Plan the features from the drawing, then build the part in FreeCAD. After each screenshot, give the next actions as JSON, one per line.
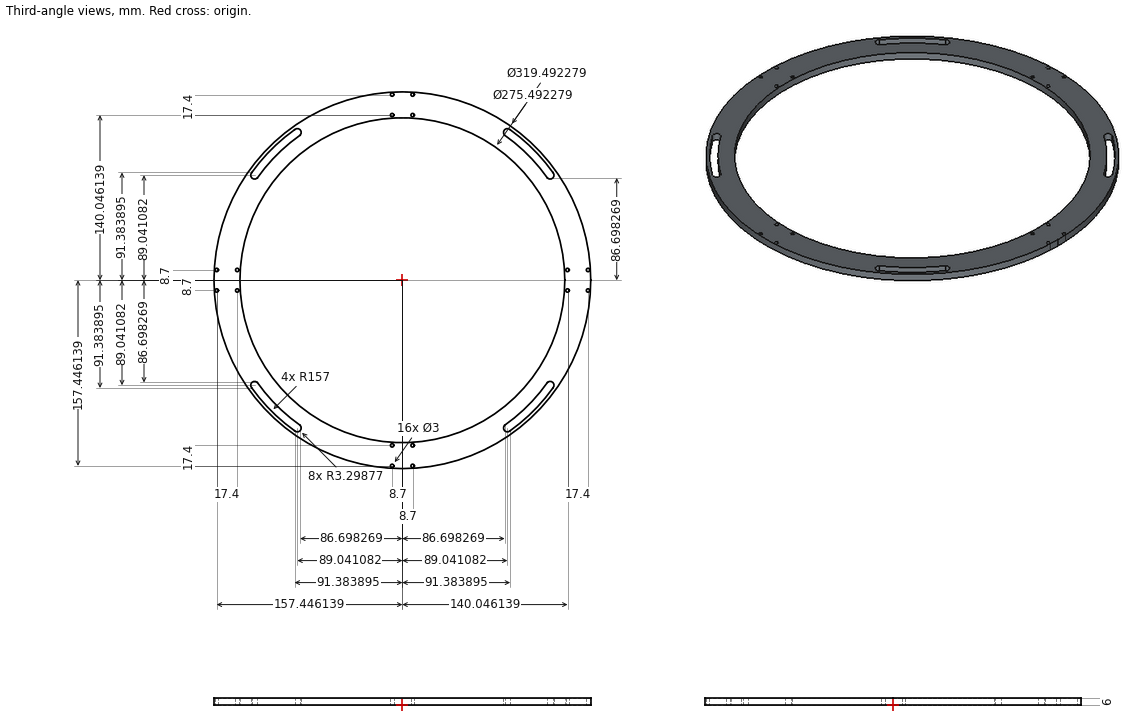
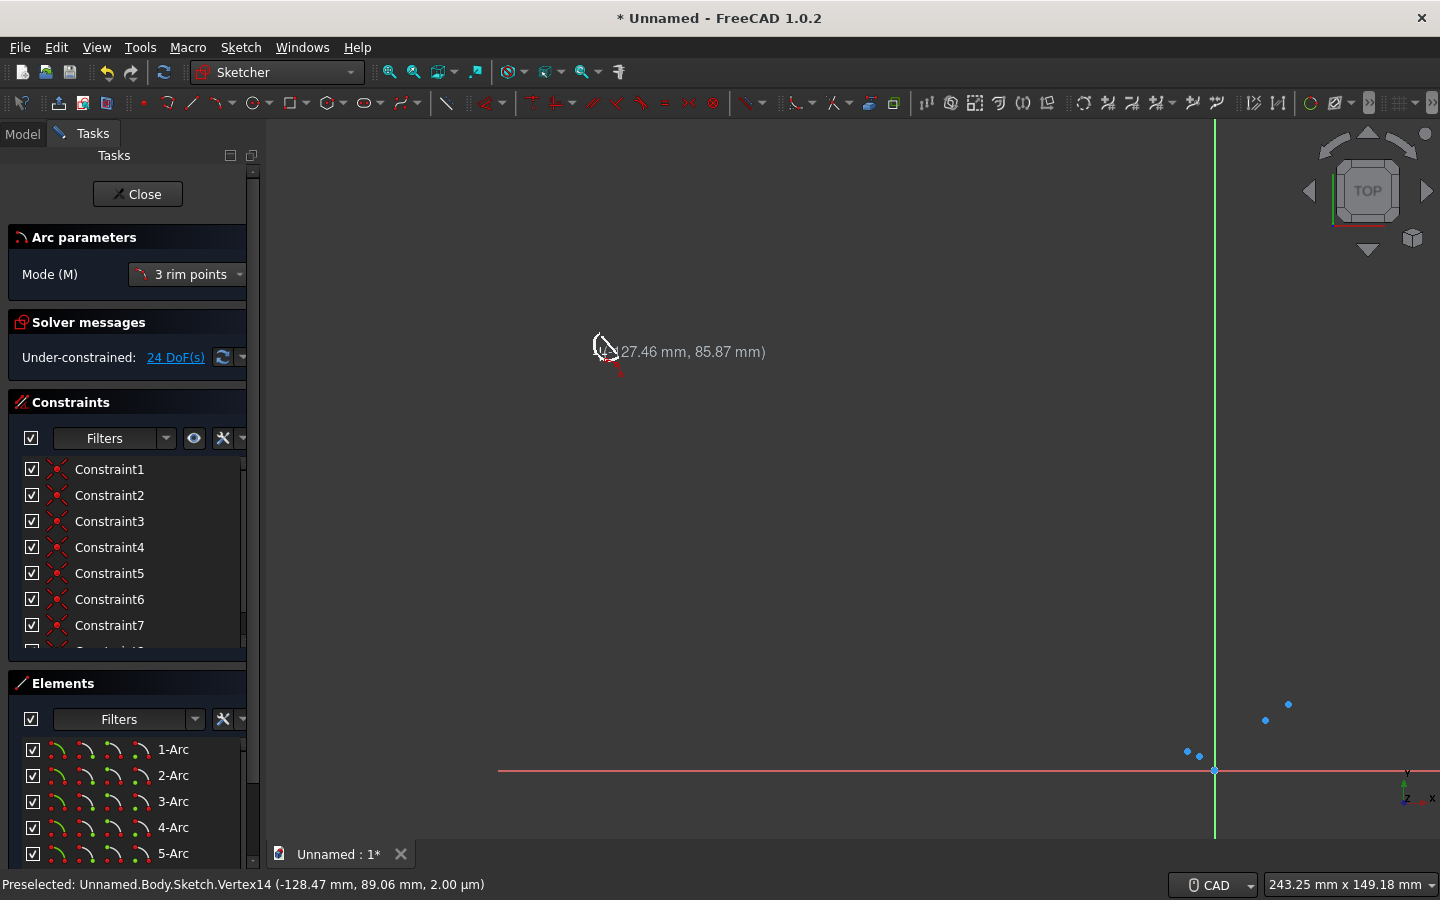
{"action": "left_click", "coordinate": [598, 352]}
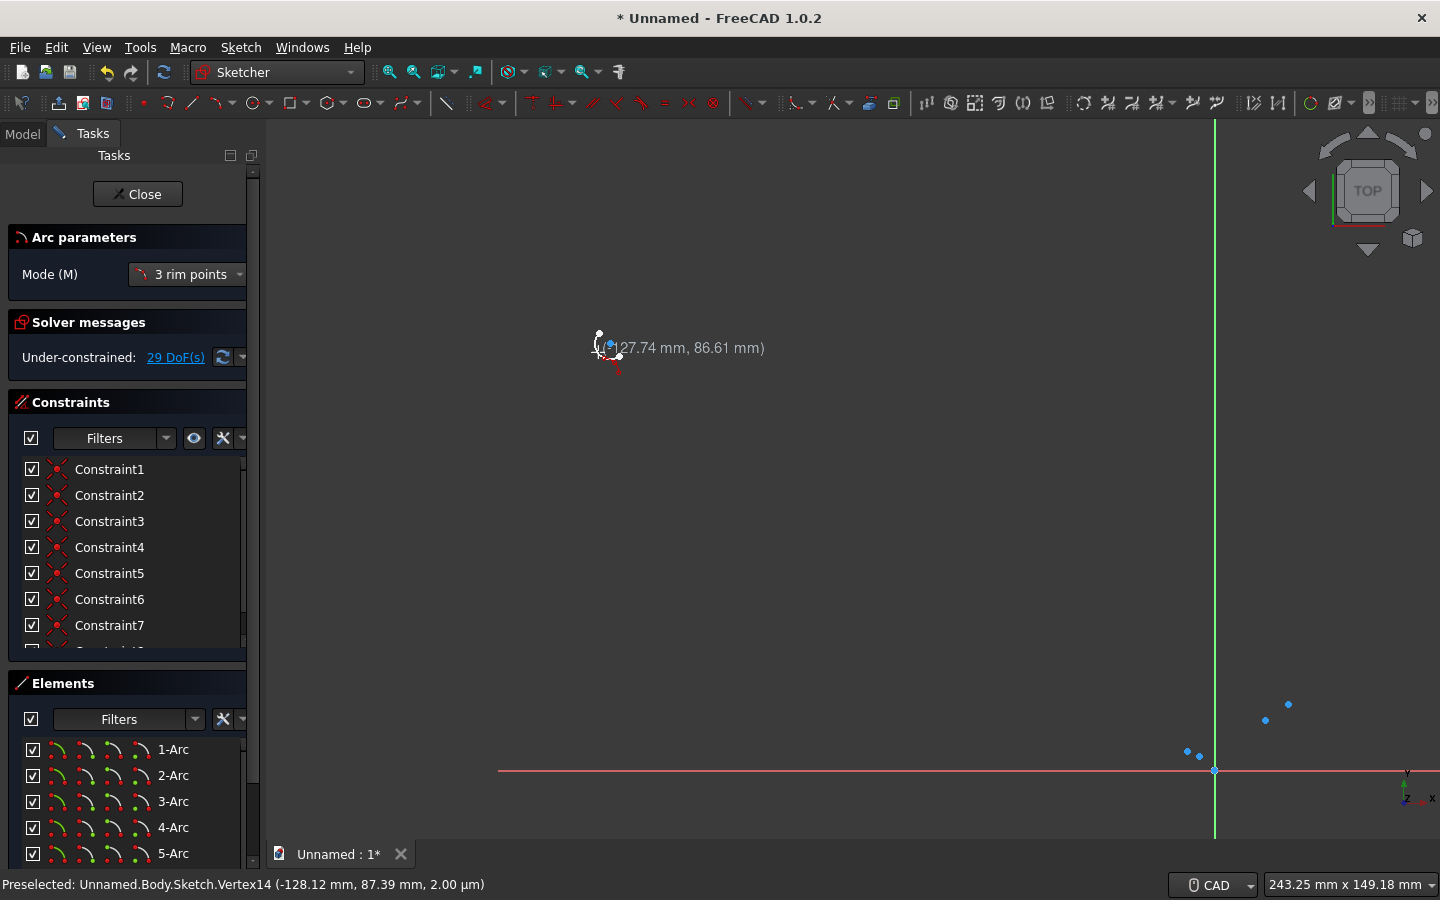
{"action": "left_click", "coordinate": [599, 333]}
{"action": "left_click", "coordinate": [773, 155]}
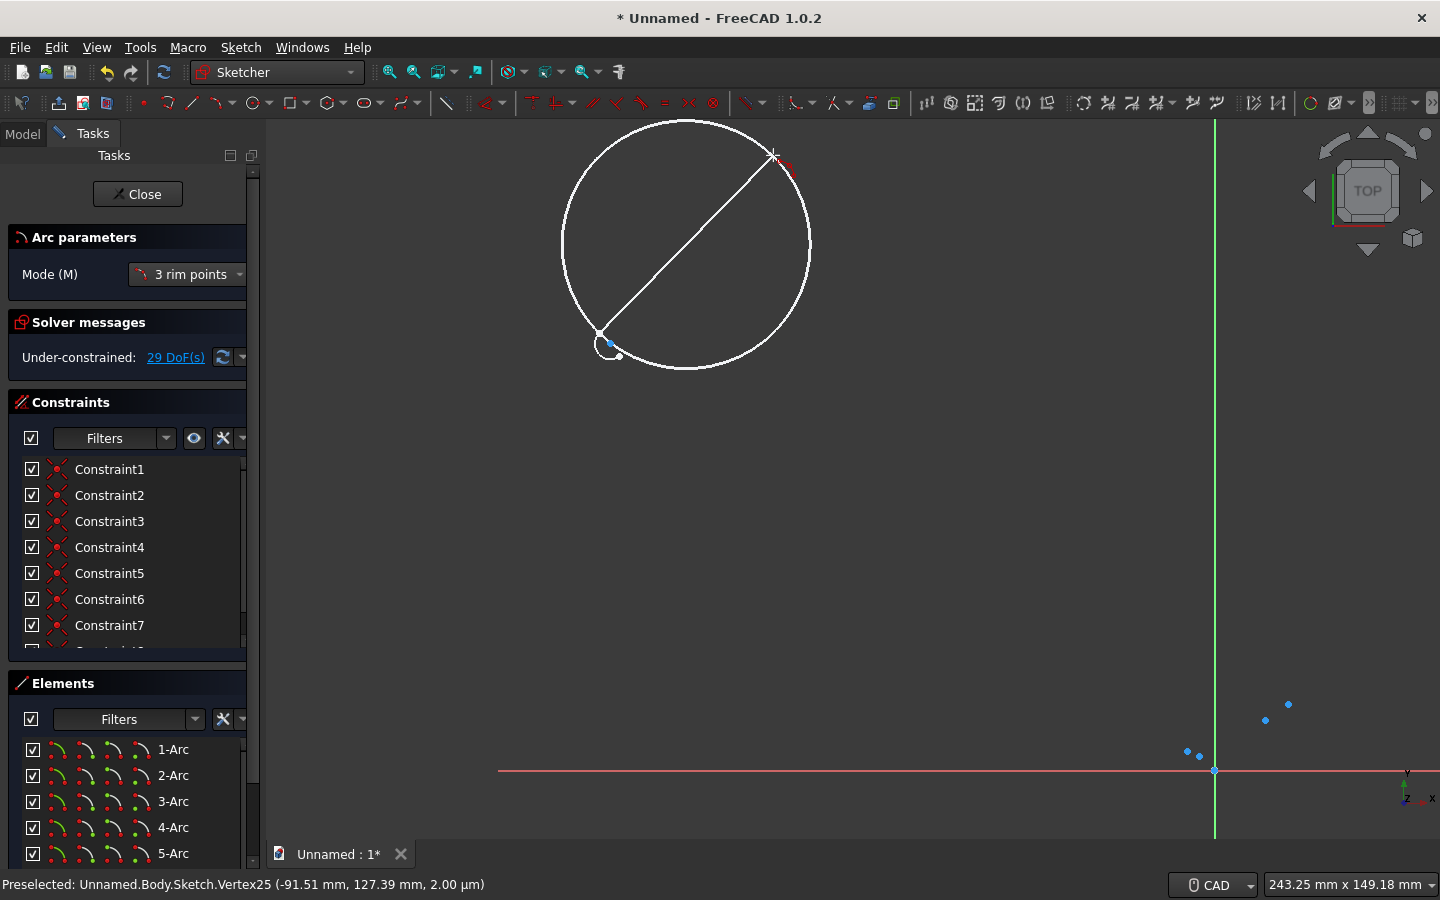
{"action": "scroll", "coordinate": [679, 235], "scroll_direction": "up", "scroll_amount": 3}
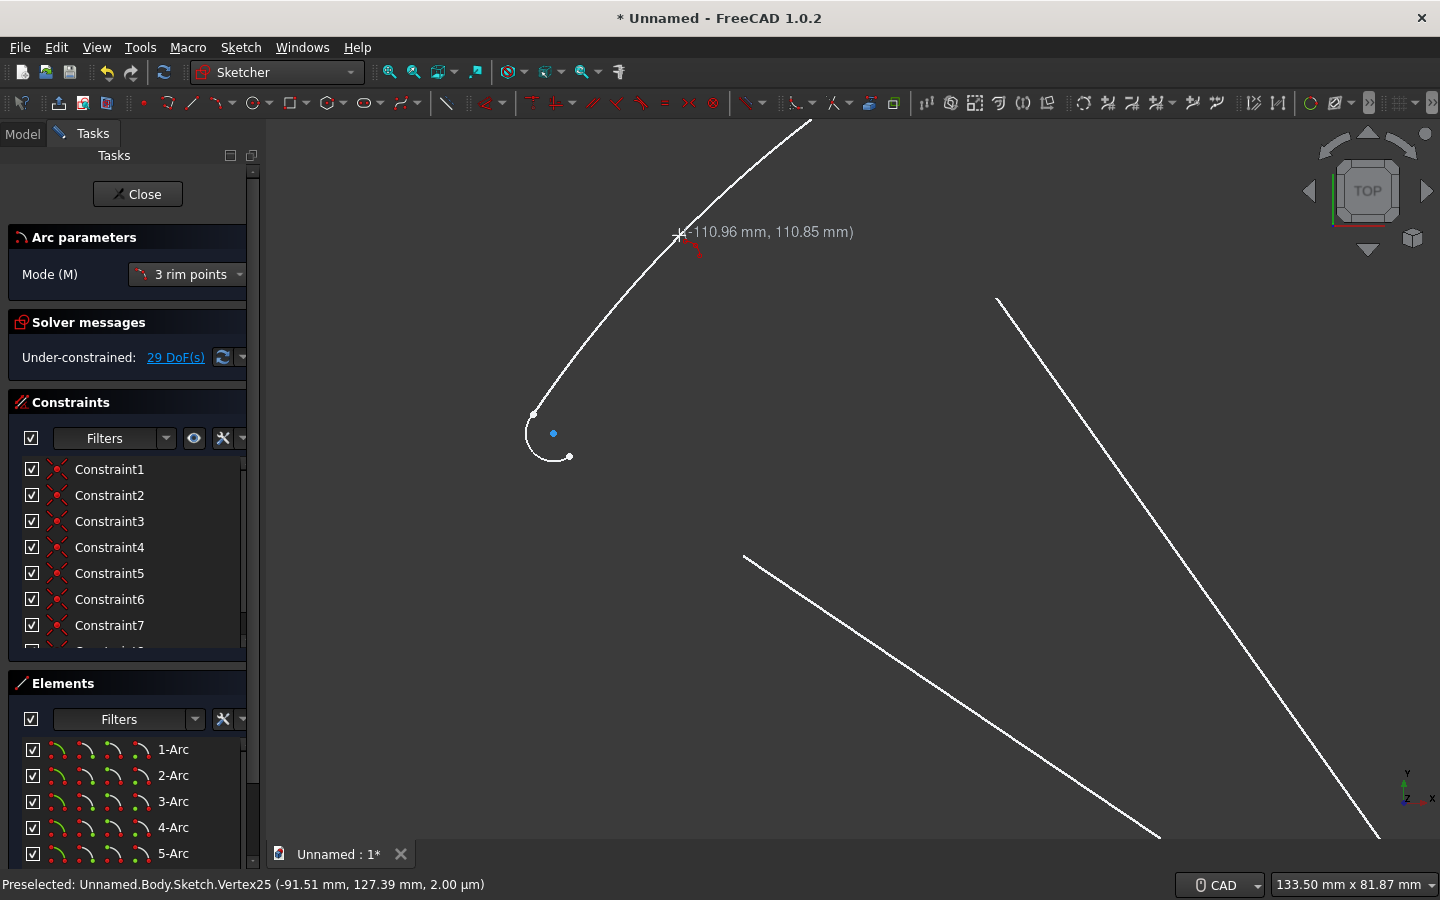
{"action": "left_click", "coordinate": [678, 235]}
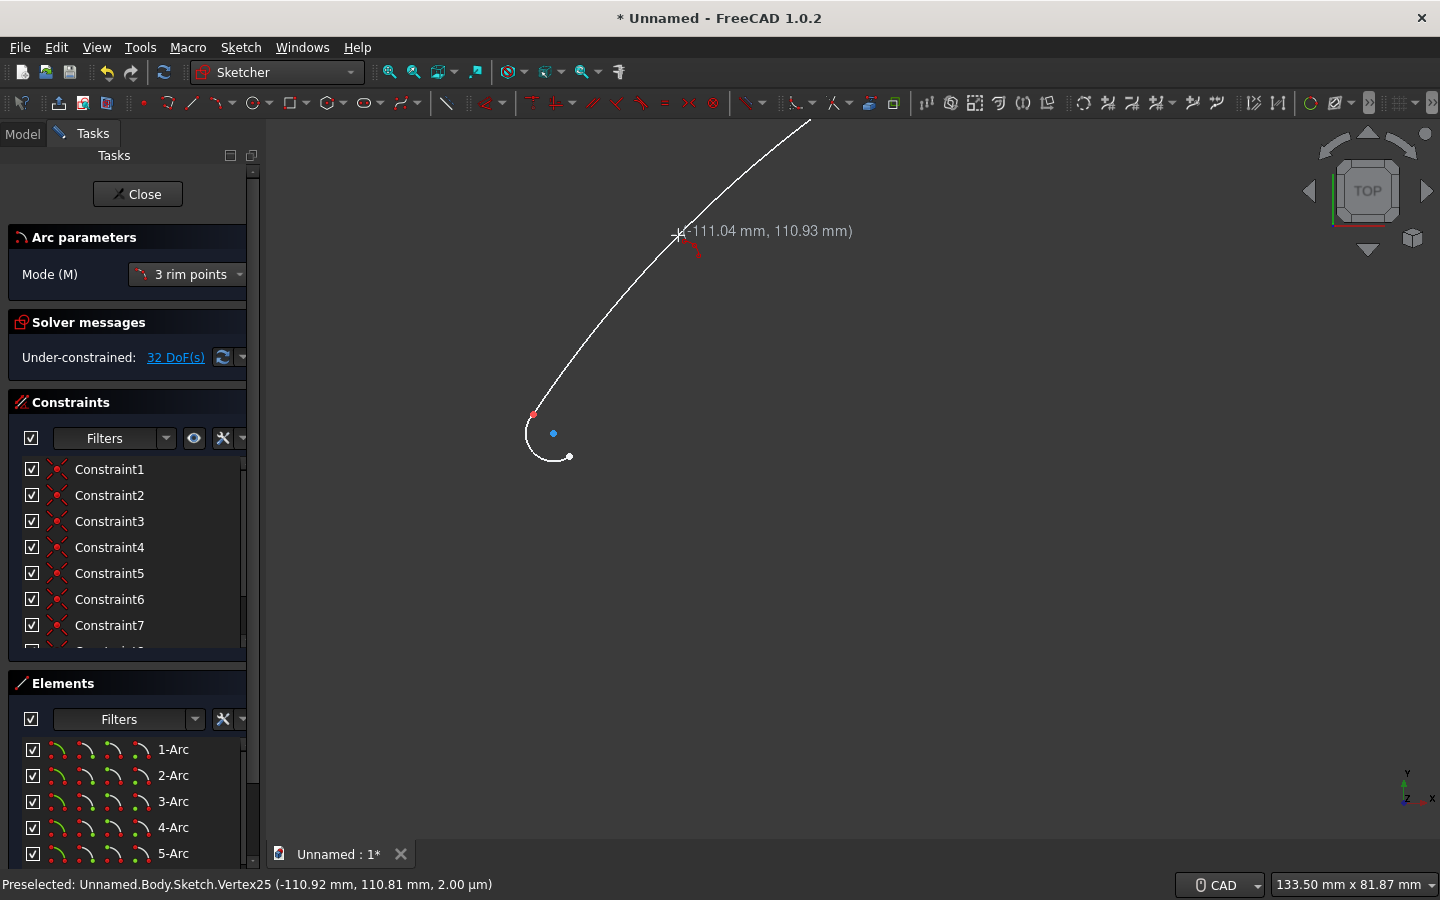
{"action": "scroll", "coordinate": [612, 334], "scroll_direction": "down", "scroll_amount": 9}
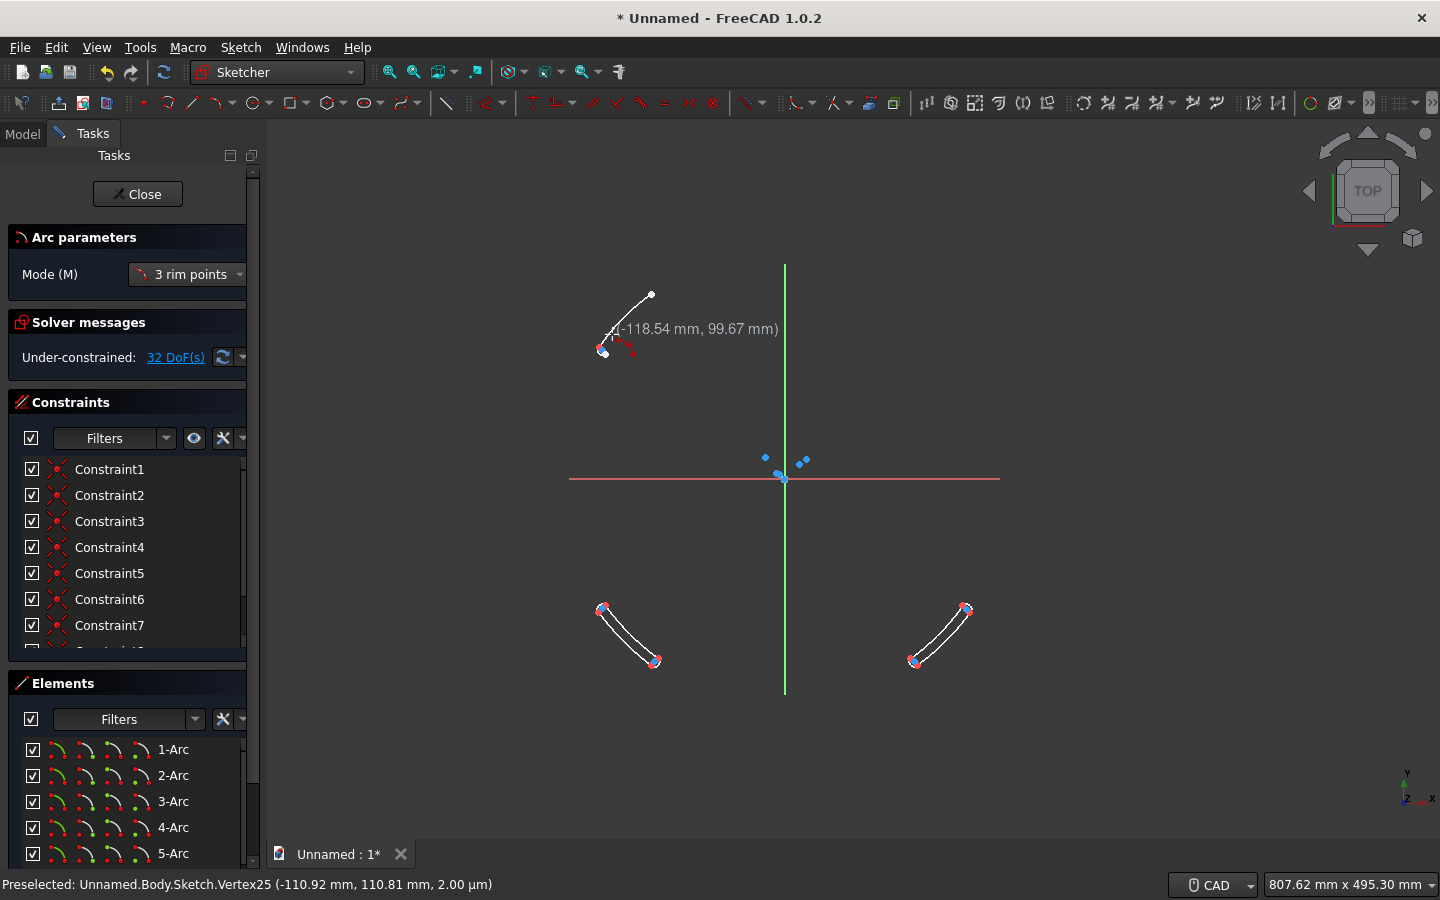
{"action": "left_click", "coordinate": [652, 294]}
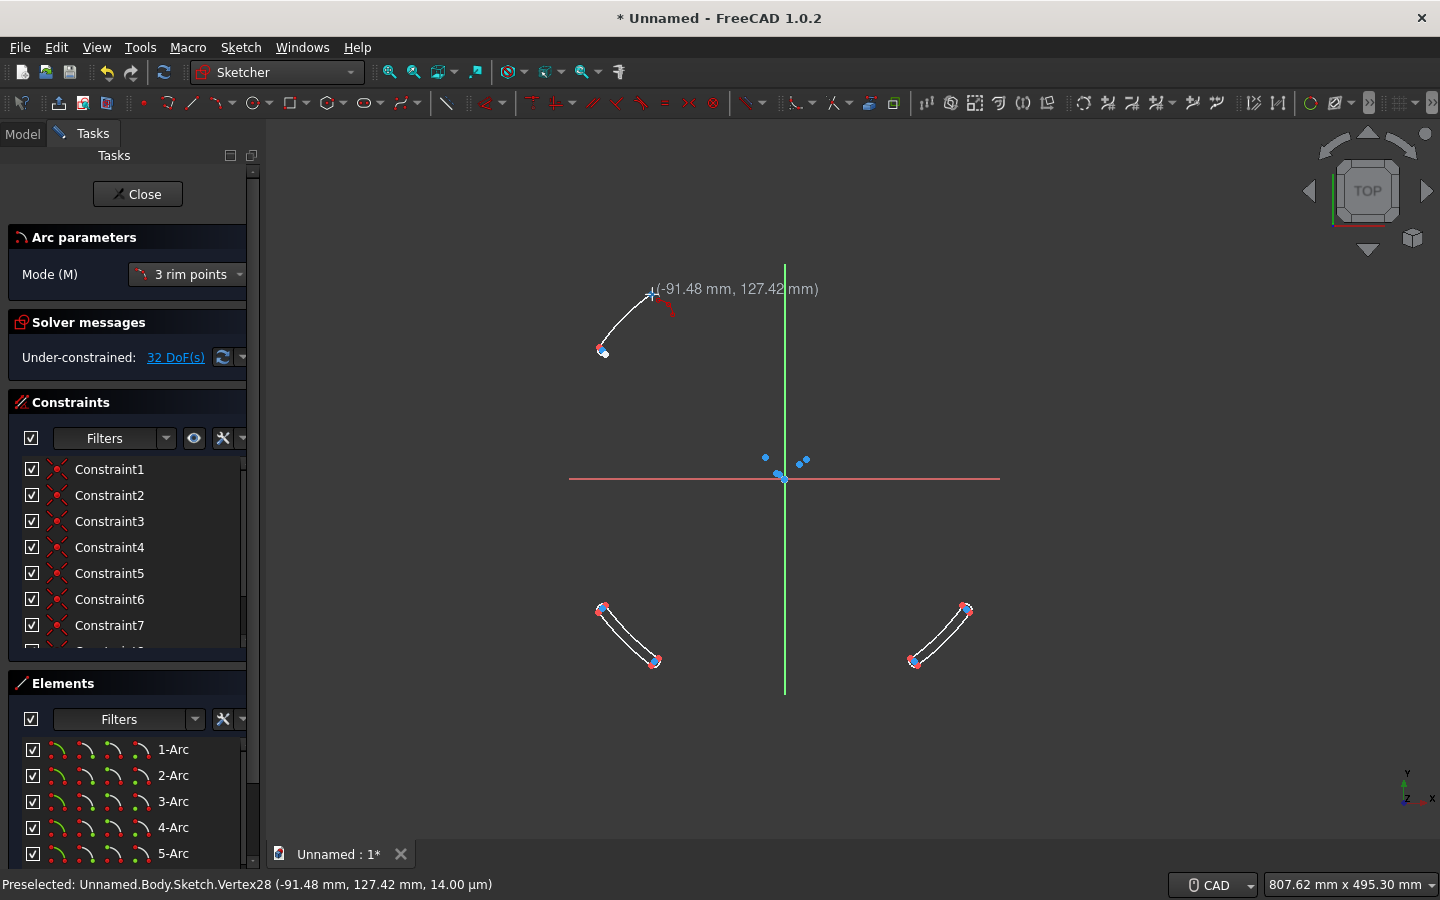
{"action": "scroll", "coordinate": [659, 300], "scroll_direction": "up", "scroll_amount": 3}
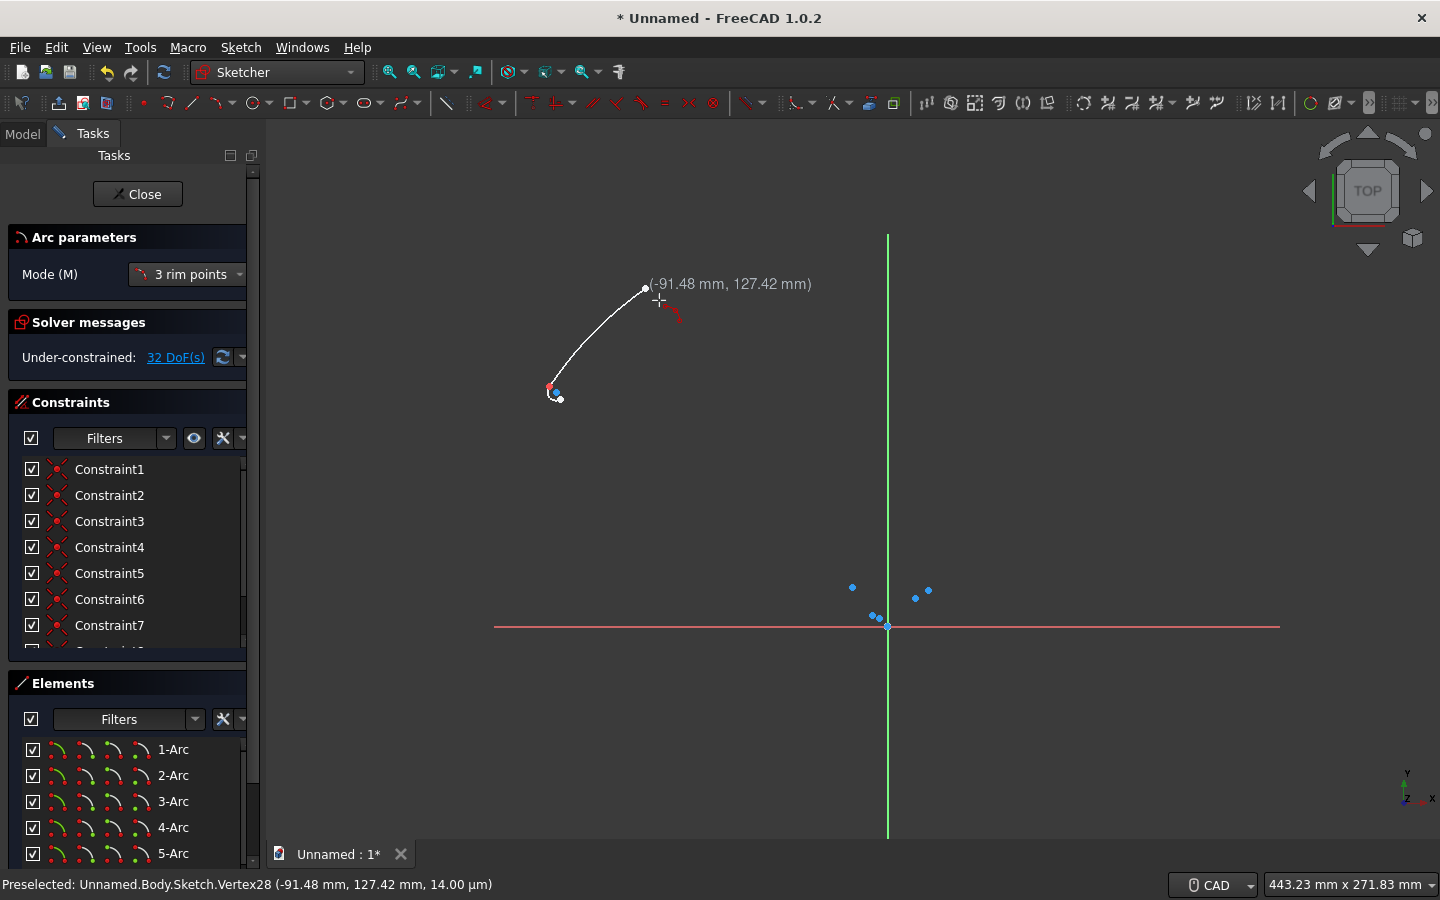
{"action": "left_click", "coordinate": [658, 301]}